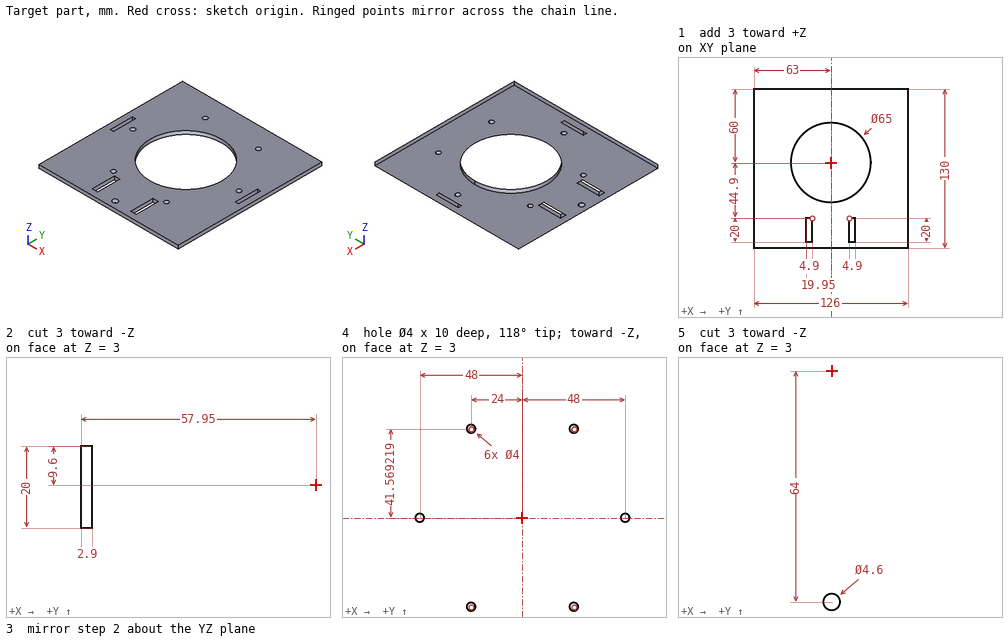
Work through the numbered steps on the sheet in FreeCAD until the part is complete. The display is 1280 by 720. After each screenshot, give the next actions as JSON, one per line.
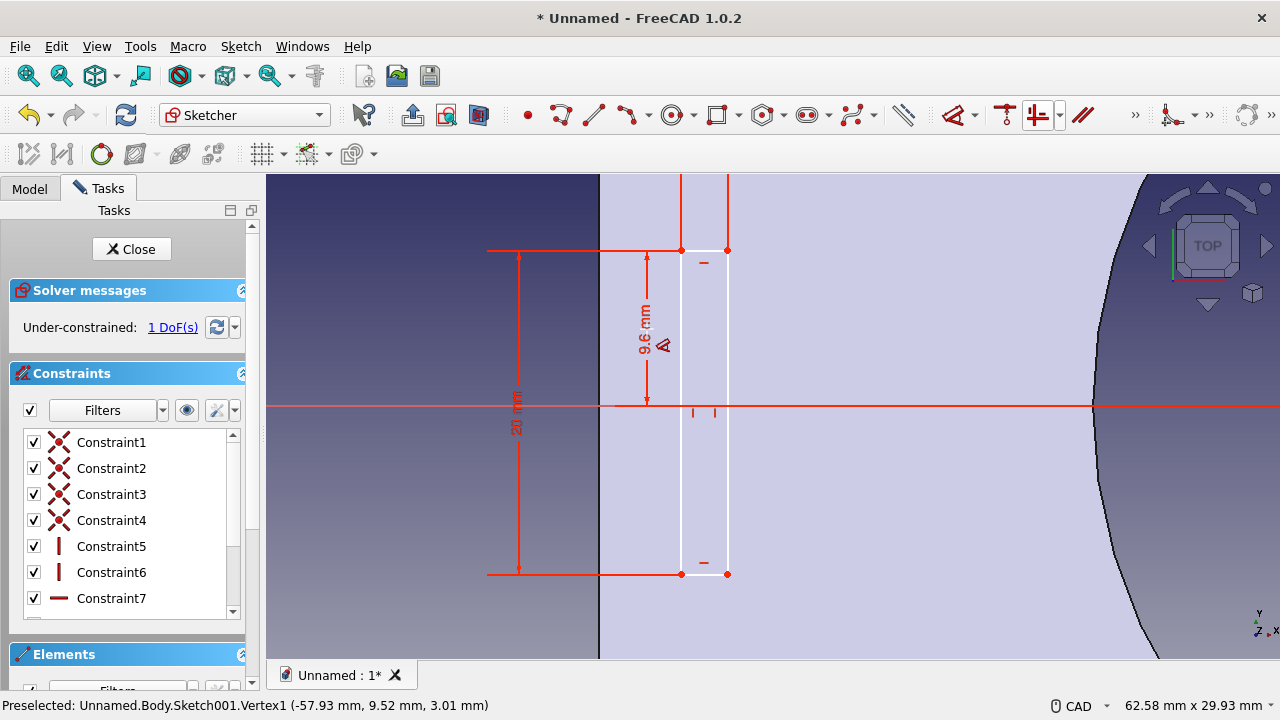
{"action": "left_click", "coordinate": [681, 251]}
{"action": "left_click", "coordinate": [898, 217]}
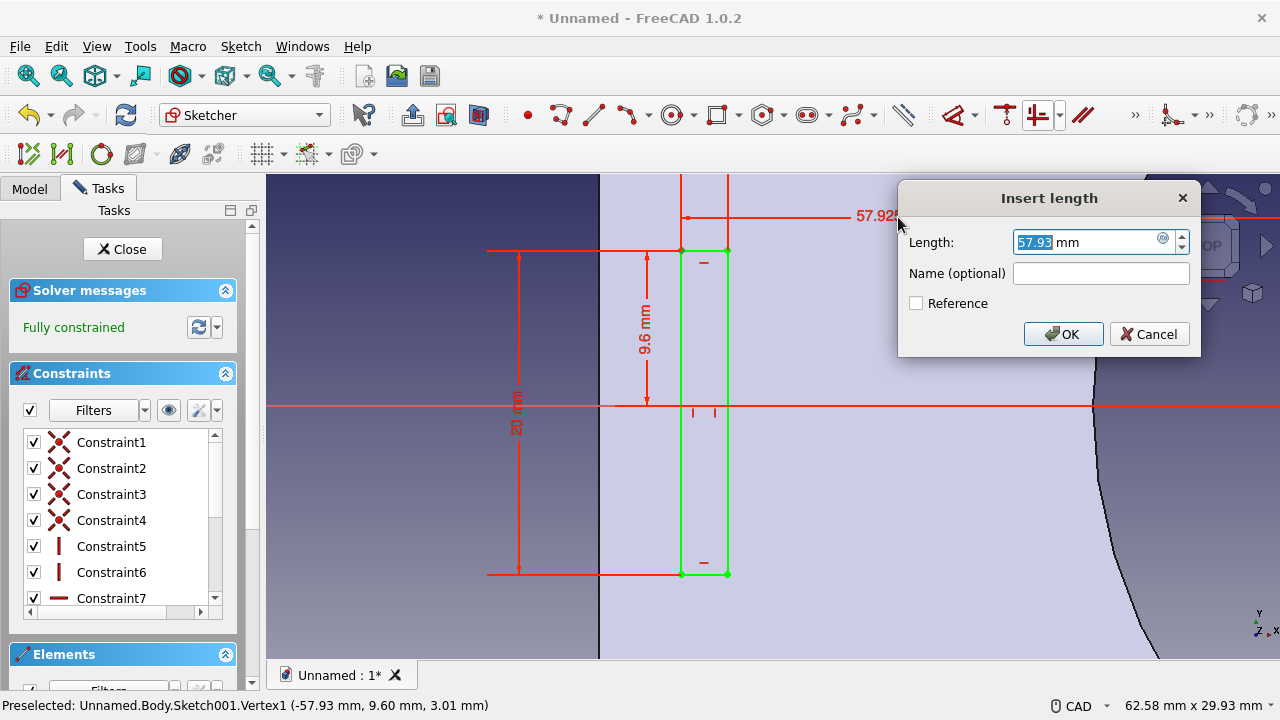
{"action": "type", "text": "57.95"}
{"action": "key", "text": "Return"}
{"action": "key", "text": "Escape"}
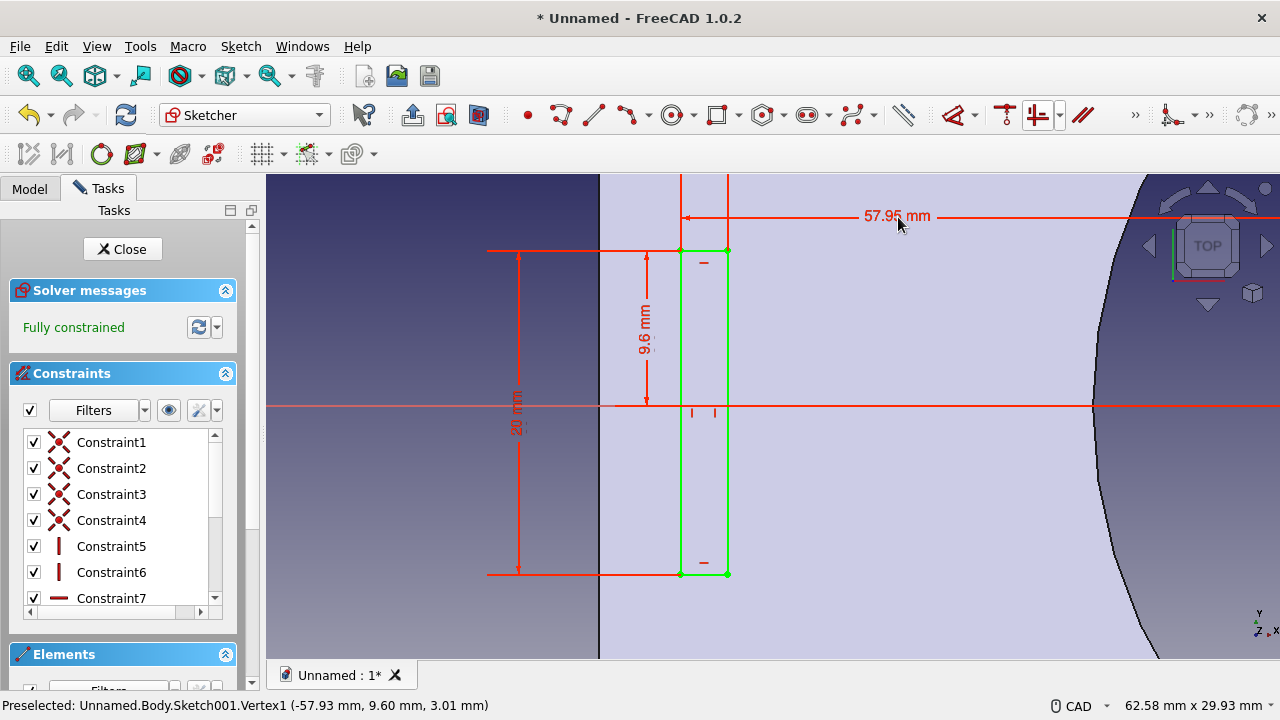
{"action": "left_click", "coordinate": [123, 249]}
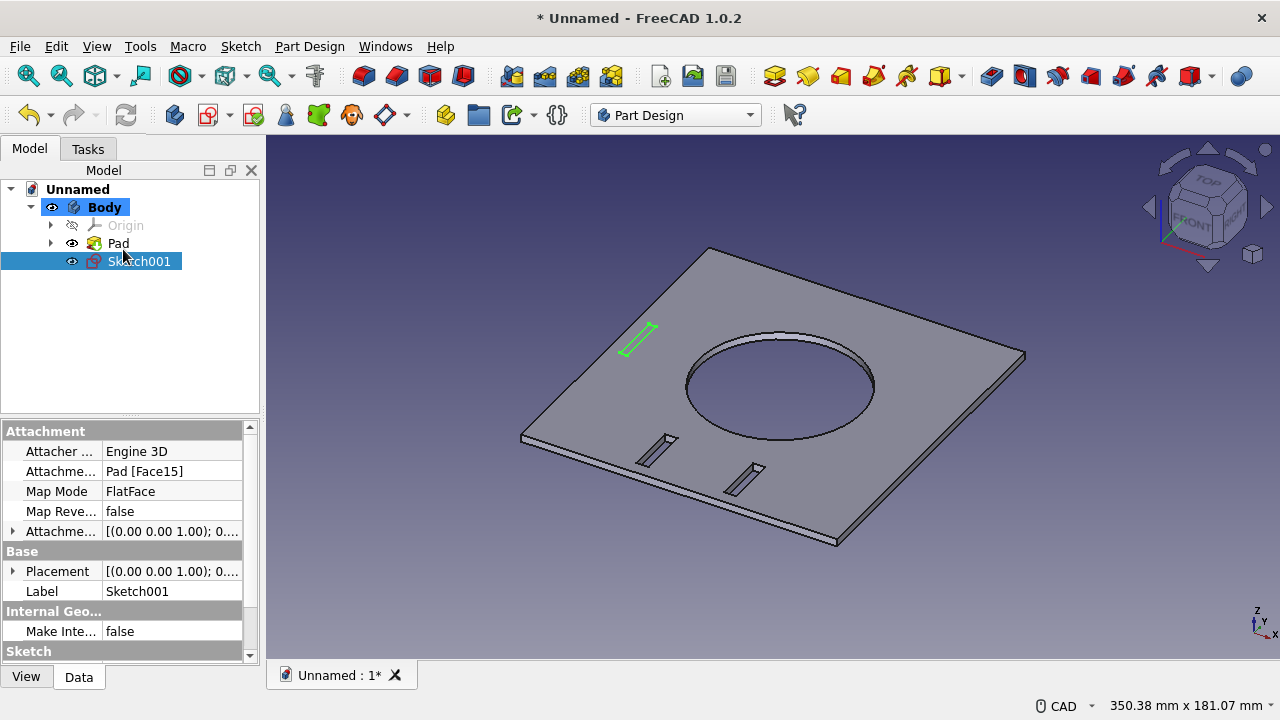
{"action": "left_click", "coordinate": [992, 76]}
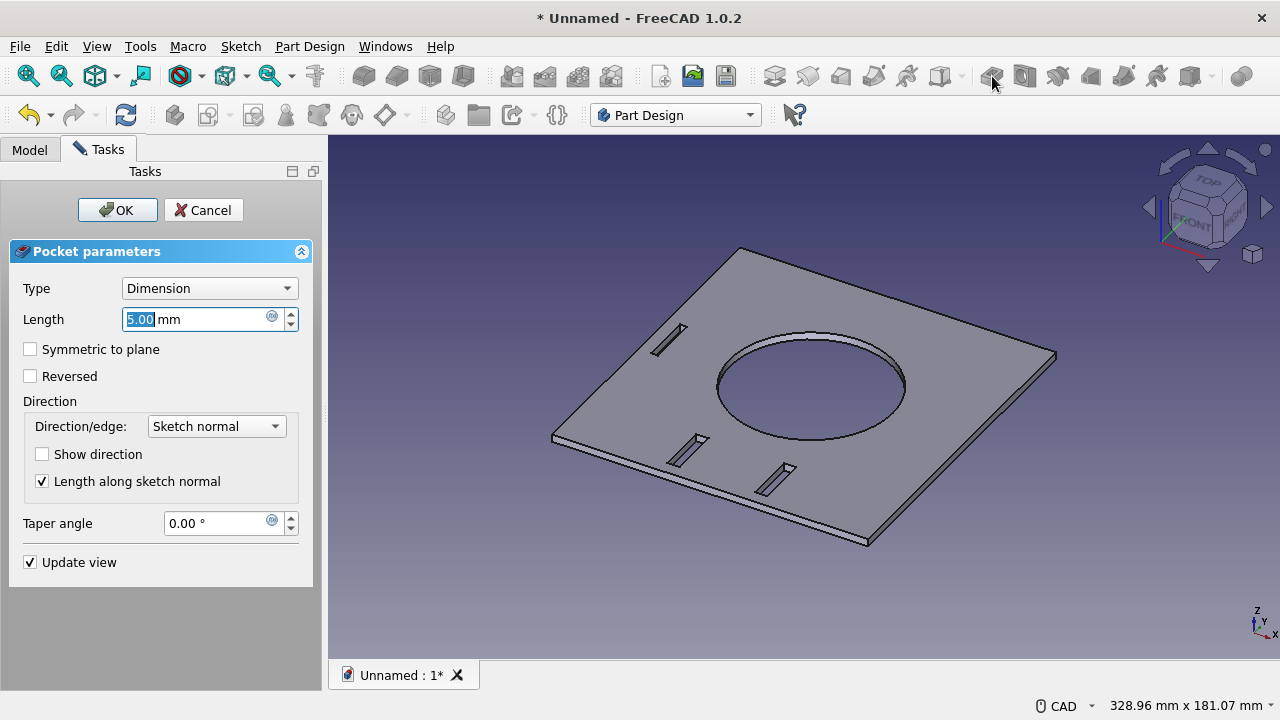
{"action": "type", "text": "3"}
{"action": "key", "text": "Tab"}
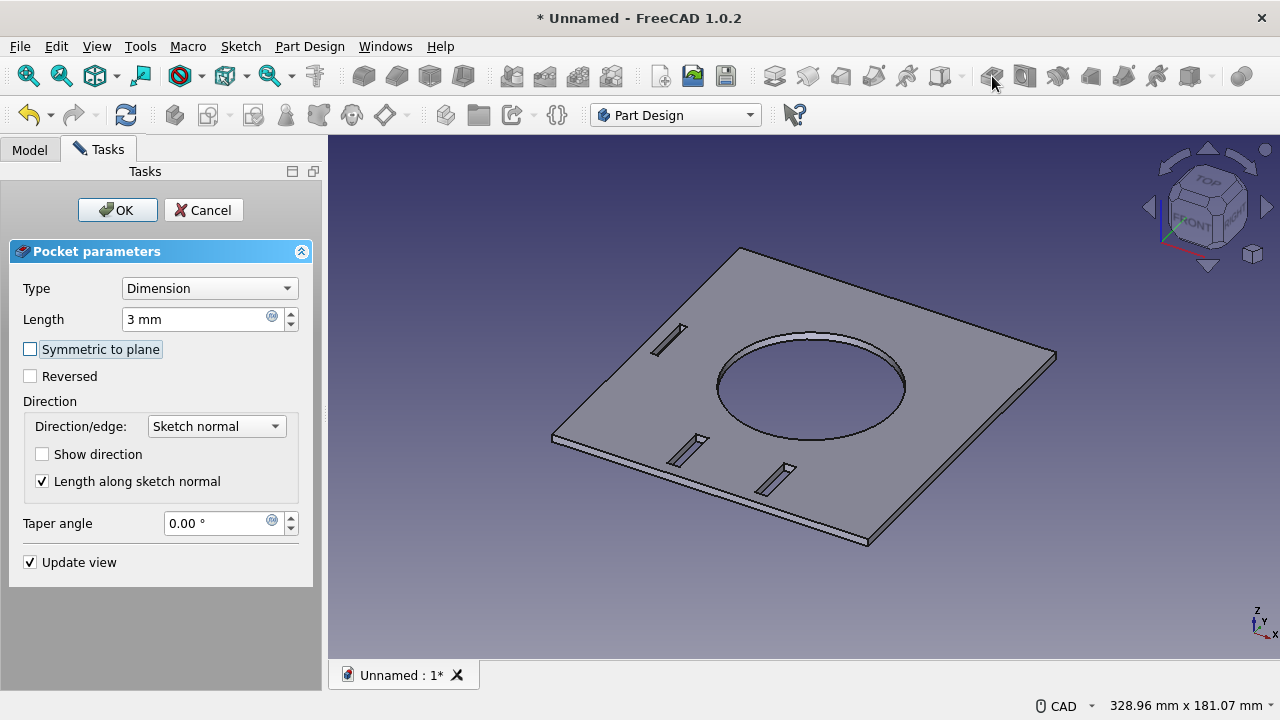
{"action": "left_click", "coordinate": [118, 210]}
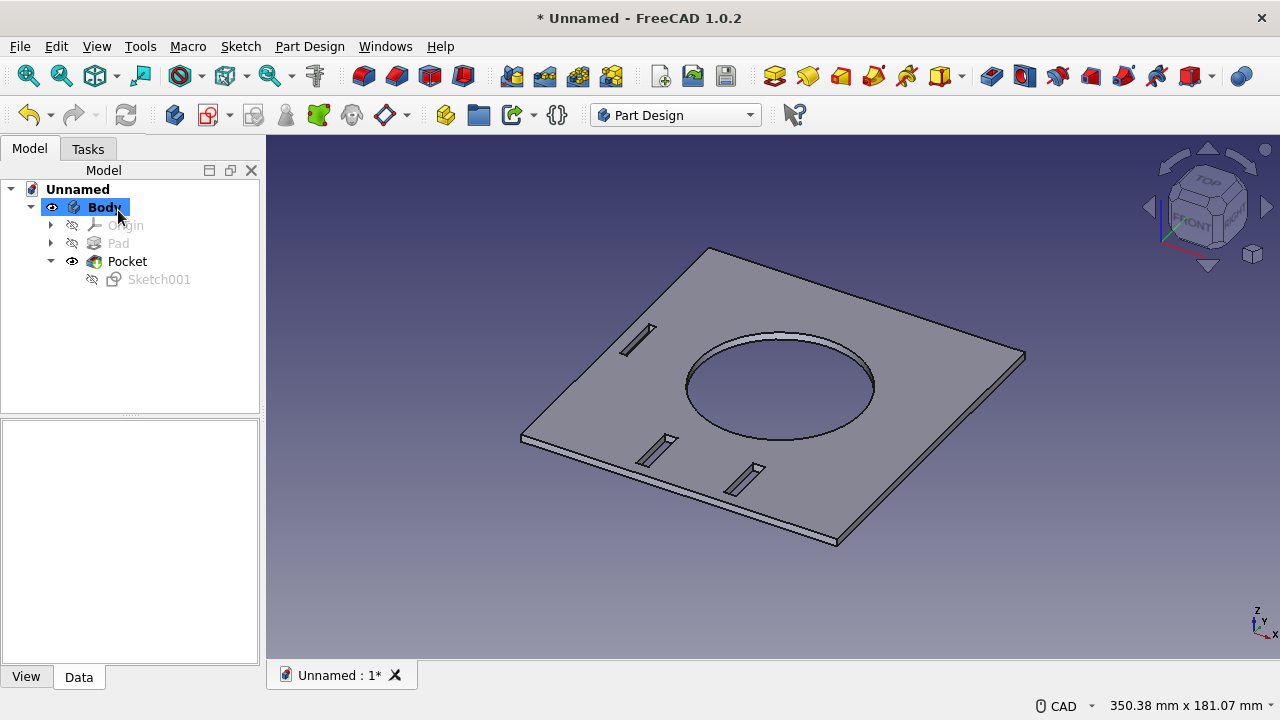
{"action": "left_click", "coordinate": [117, 261]}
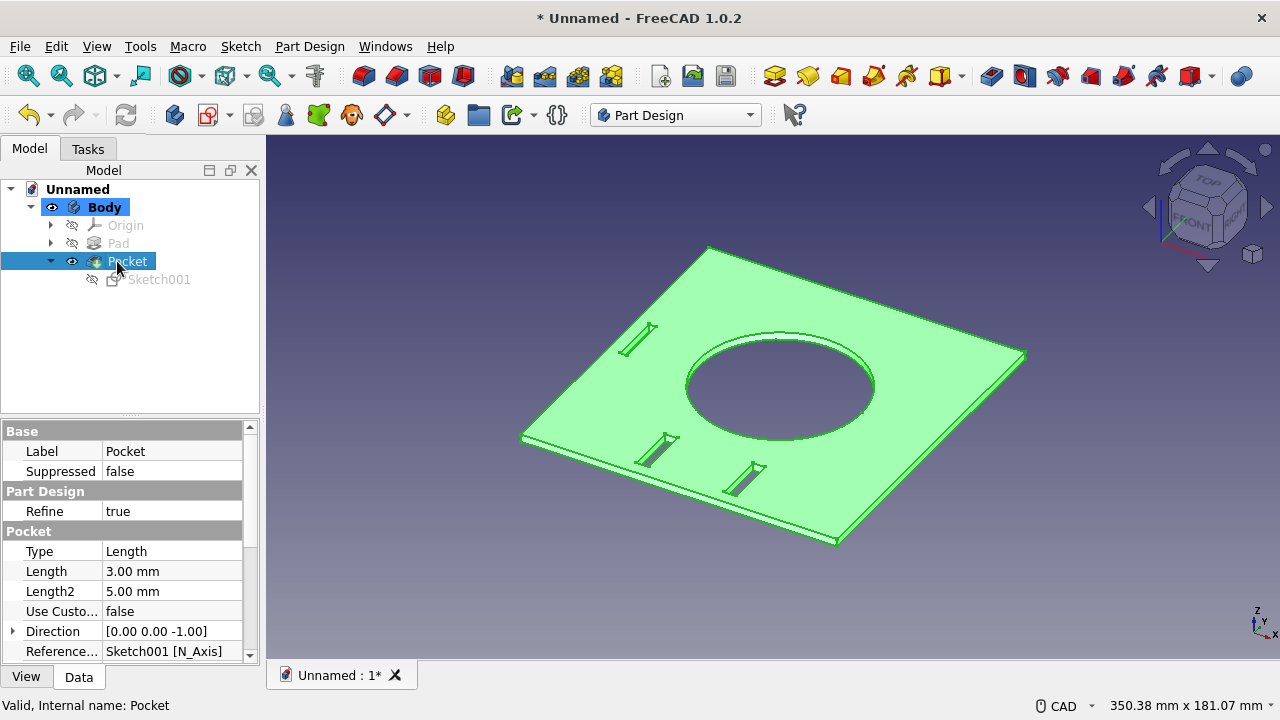
{"action": "left_click", "coordinate": [512, 76]}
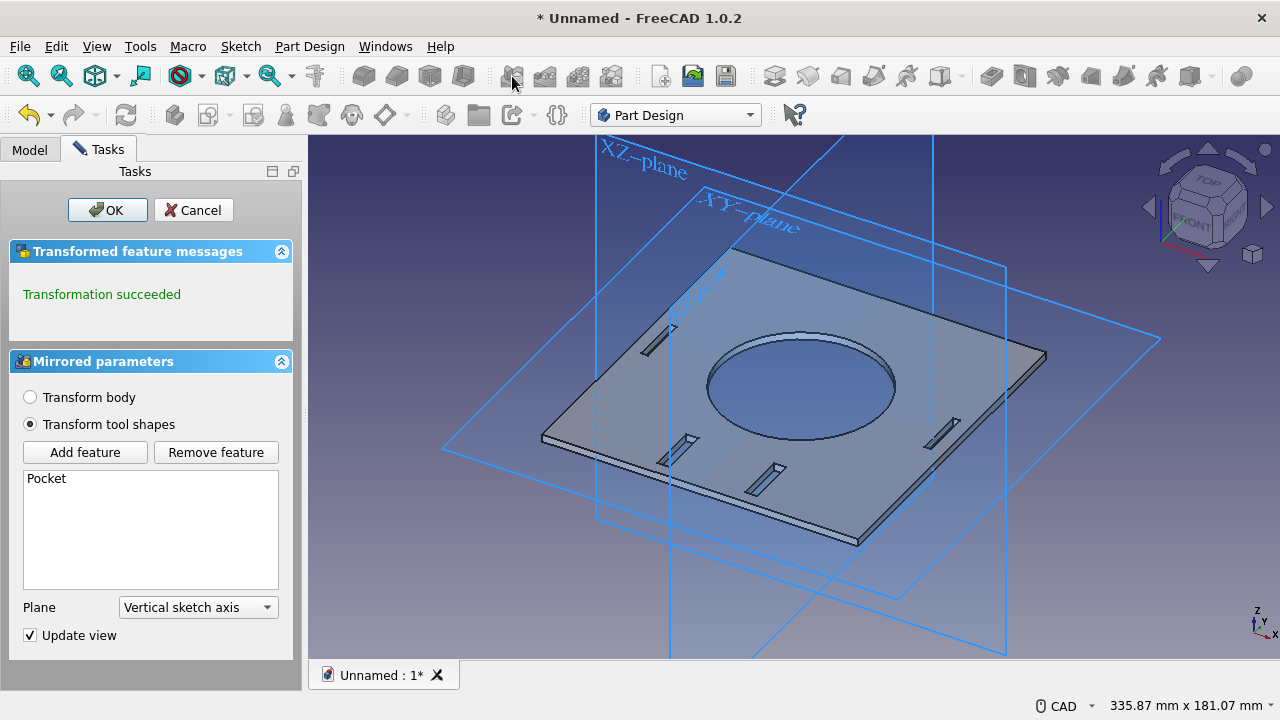
{"action": "left_click", "coordinate": [199, 608]}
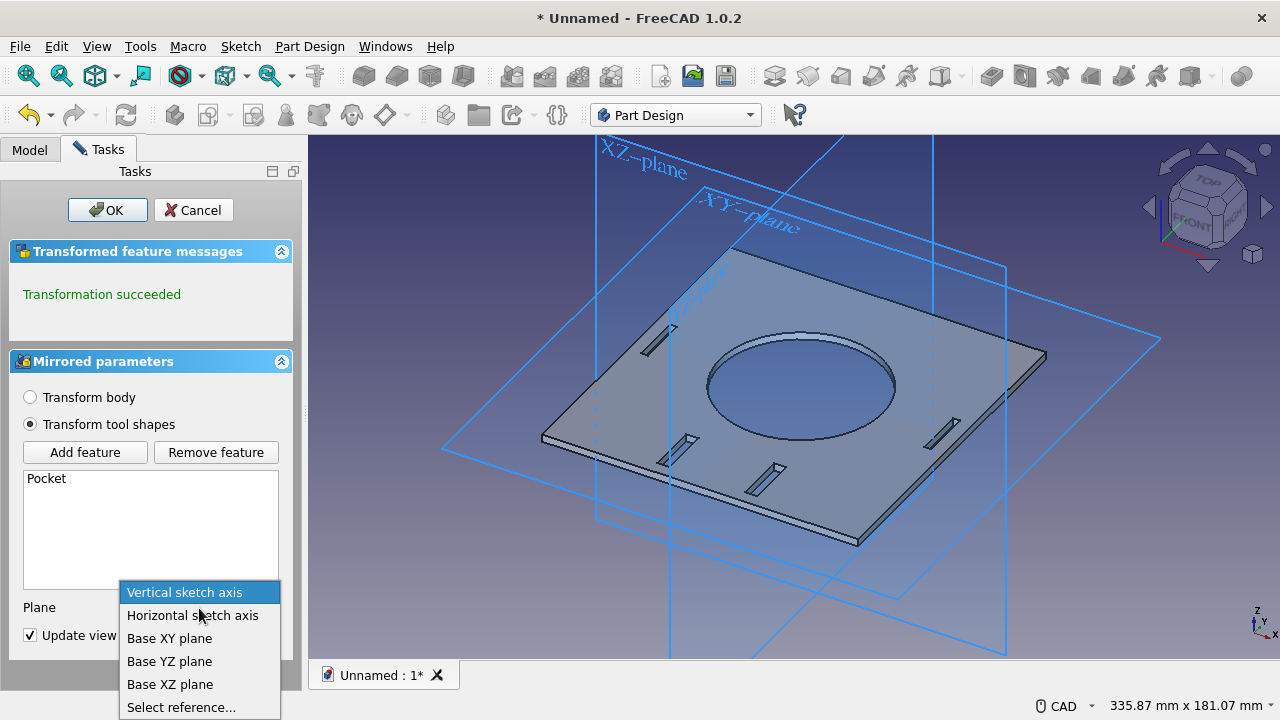
{"action": "left_click", "coordinate": [198, 662]}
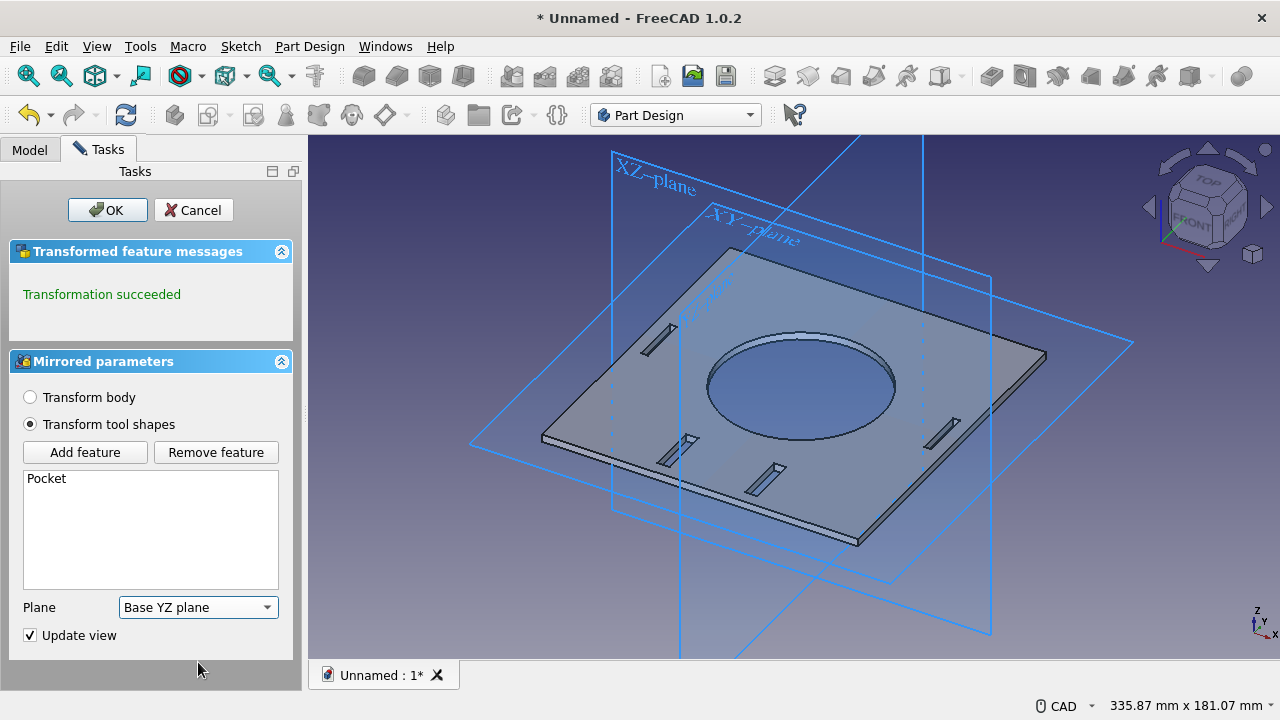
{"action": "left_click", "coordinate": [108, 210]}